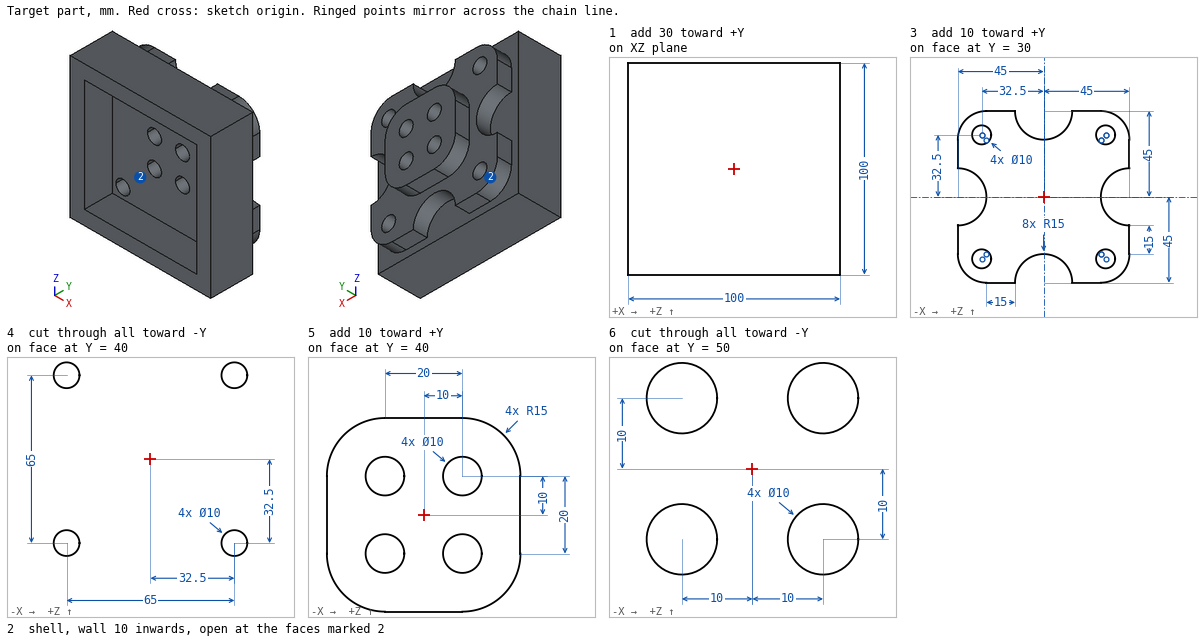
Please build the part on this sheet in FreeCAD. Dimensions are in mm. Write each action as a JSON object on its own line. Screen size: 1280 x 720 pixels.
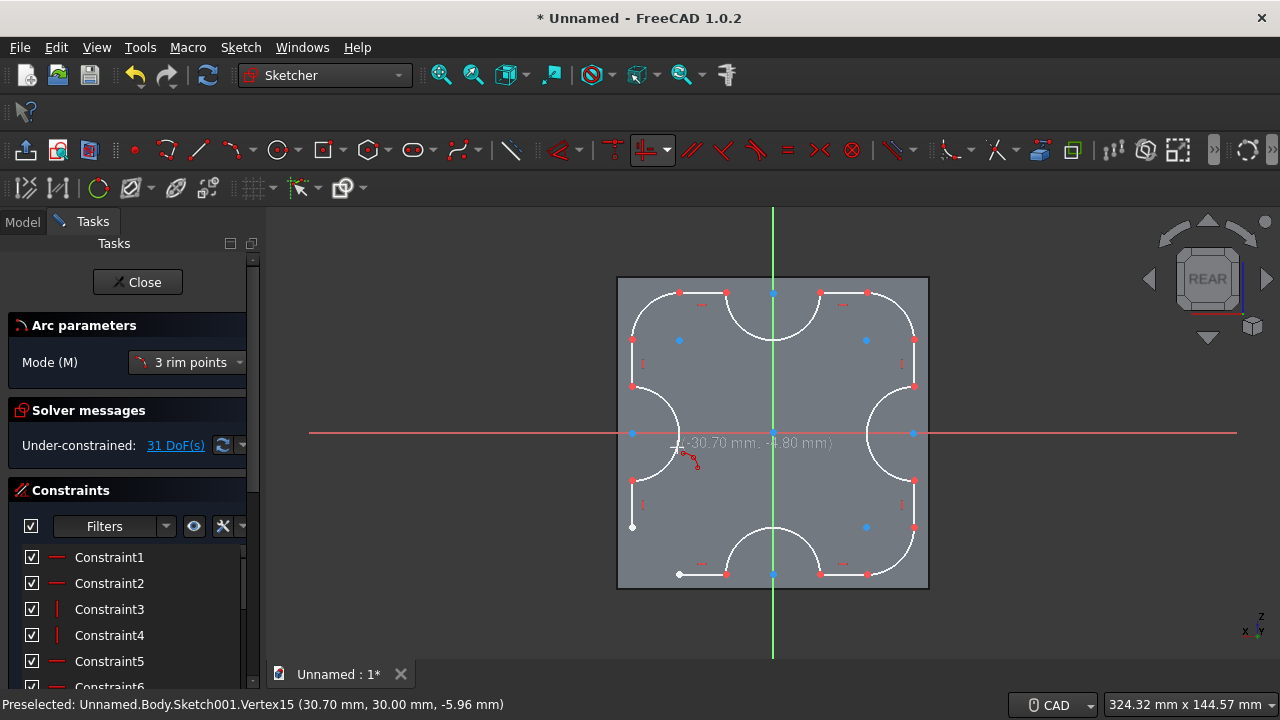
{"action": "left_click", "coordinate": [632, 528]}
{"action": "left_click", "coordinate": [679, 575]}
{"action": "left_click", "coordinate": [646, 560]}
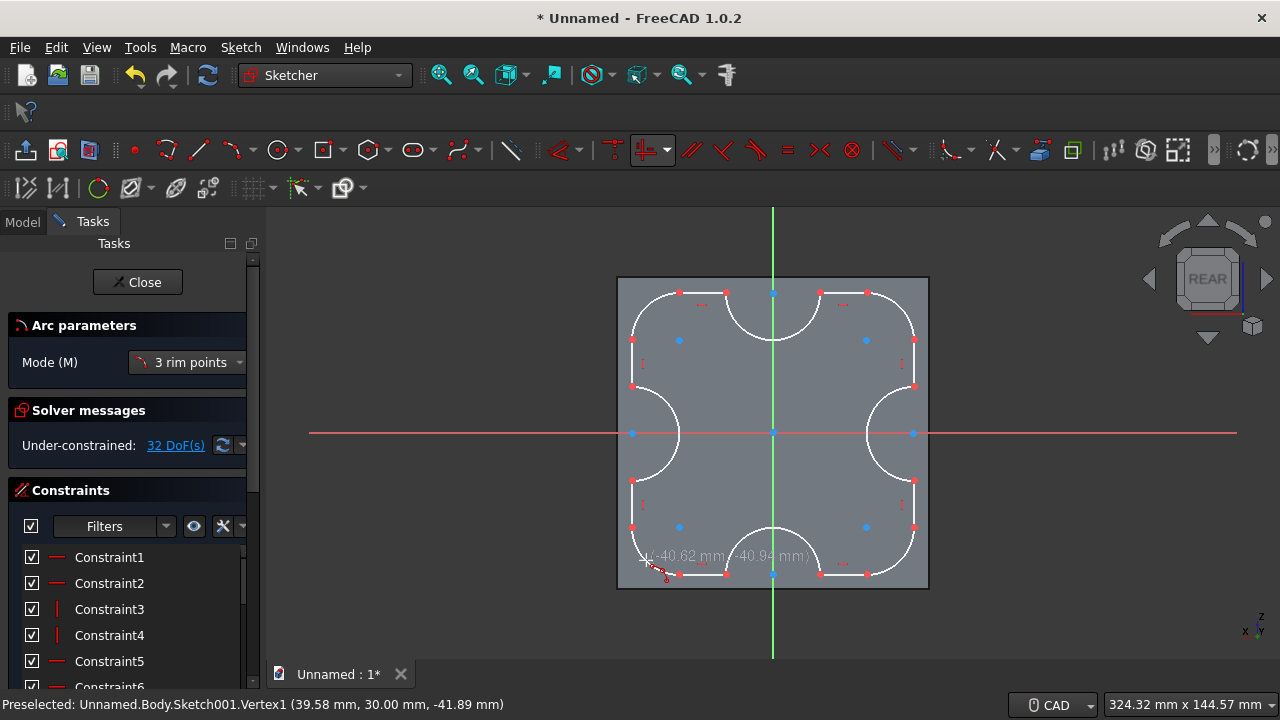
{"action": "left_click", "coordinate": [278, 150]}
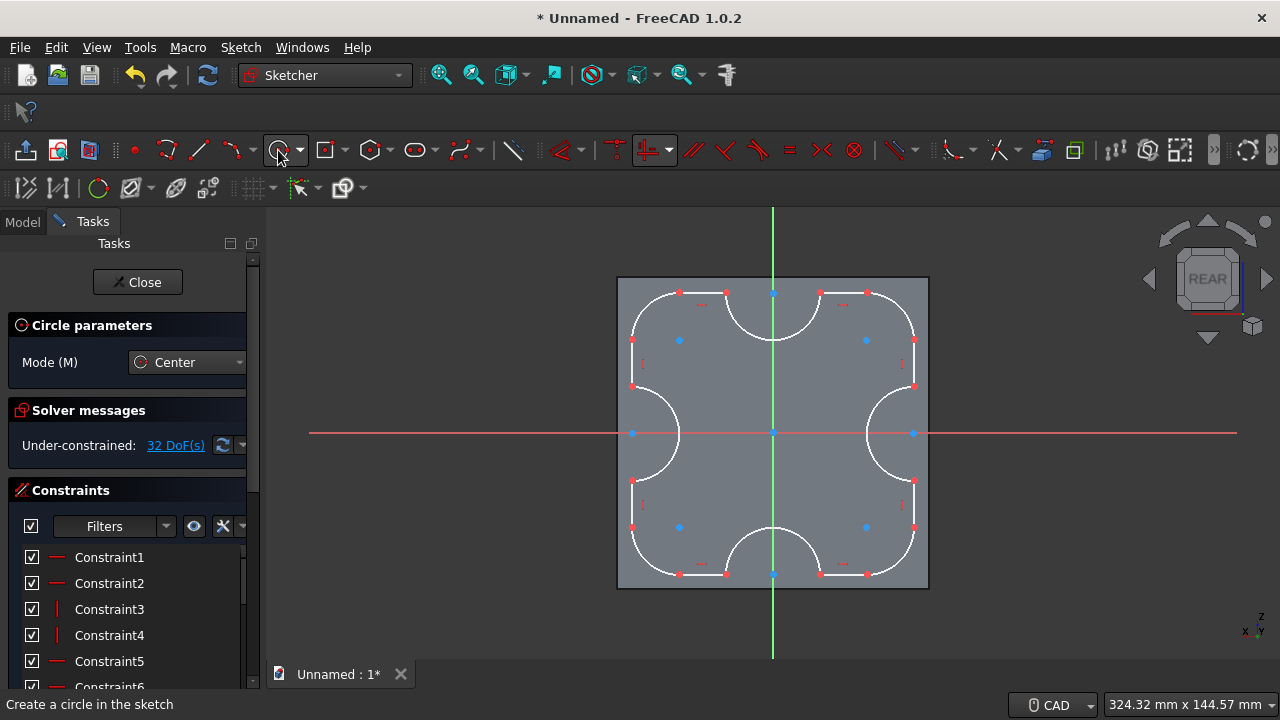
{"action": "scroll", "coordinate": [671, 331], "scroll_direction": "up", "scroll_amount": 2}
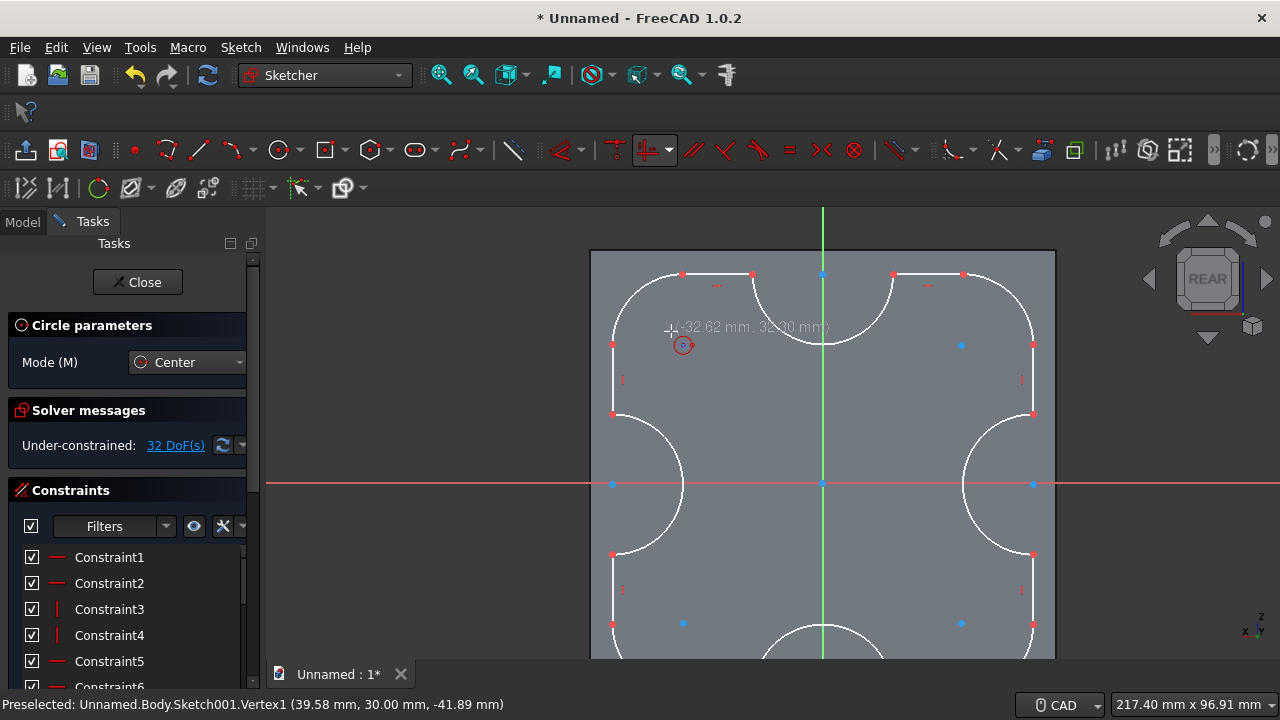
{"action": "left_click", "coordinate": [671, 331]}
{"action": "left_click", "coordinate": [688, 315]}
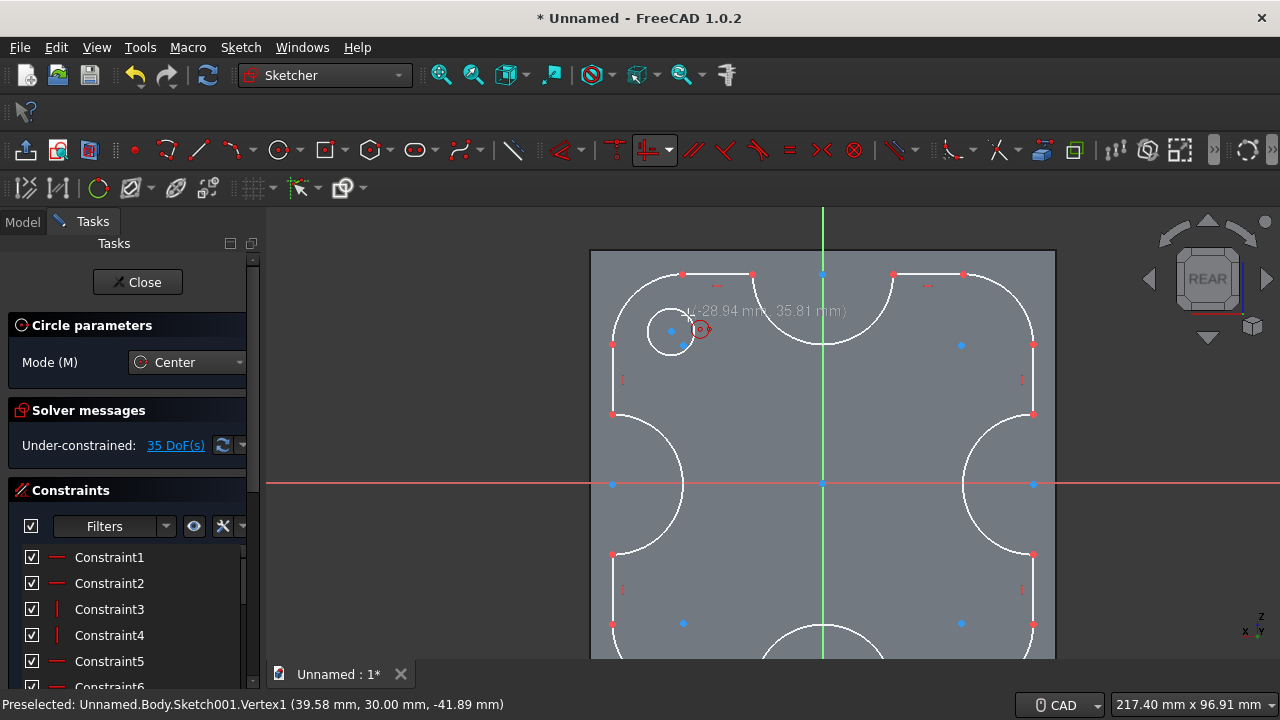
{"action": "left_click", "coordinate": [975, 331]}
{"action": "left_click", "coordinate": [991, 315]}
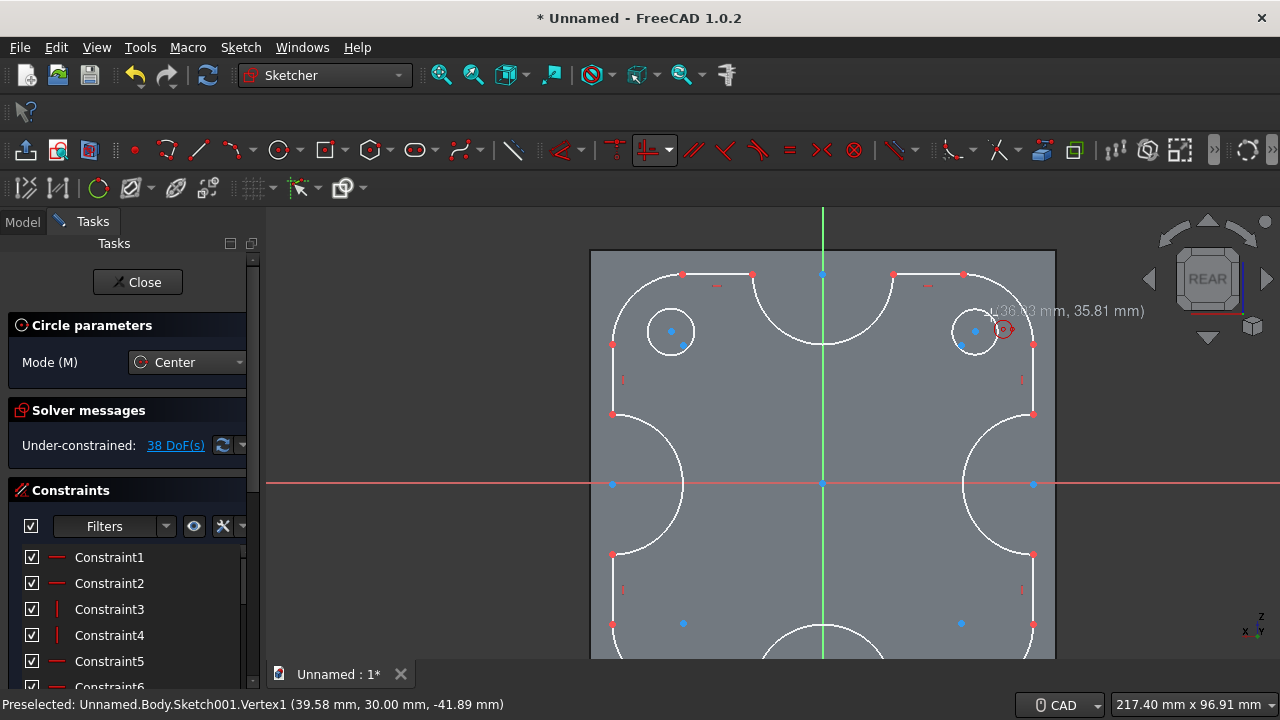
{"action": "scroll", "coordinate": [464, 331], "scroll_direction": "down", "scroll_amount": 2}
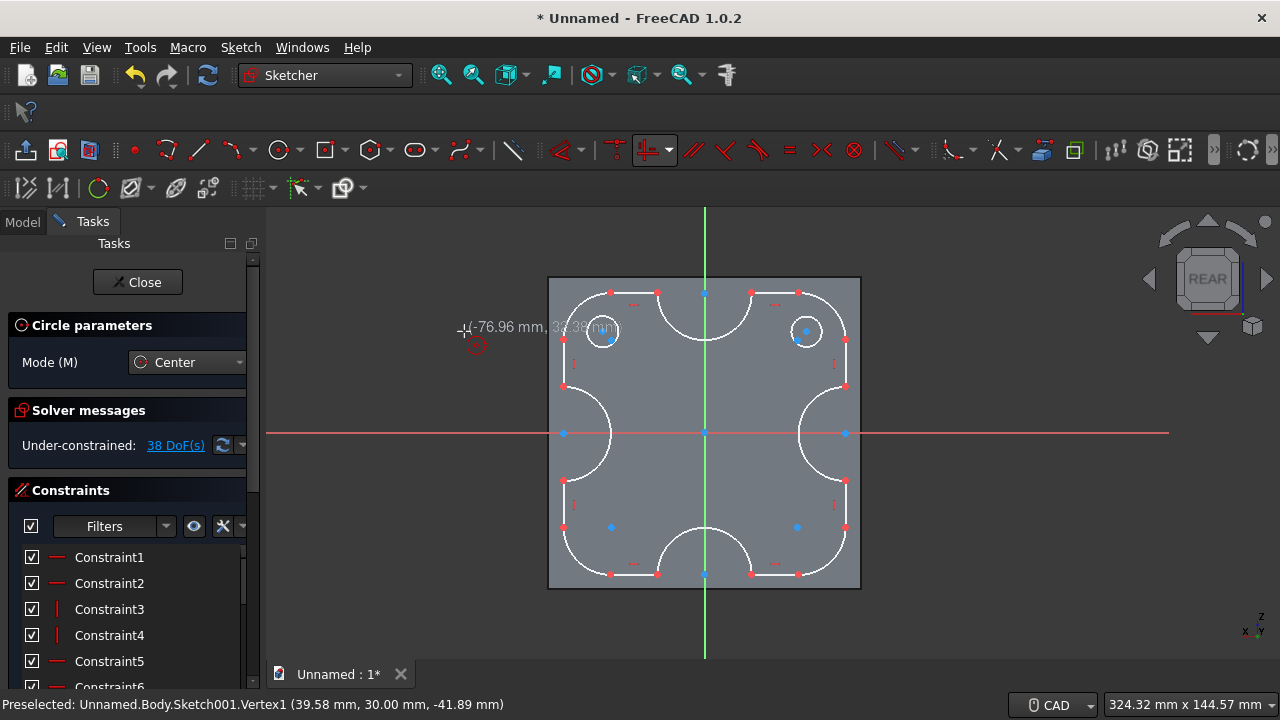
{"action": "scroll", "coordinate": [603, 535], "scroll_direction": "up", "scroll_amount": 2}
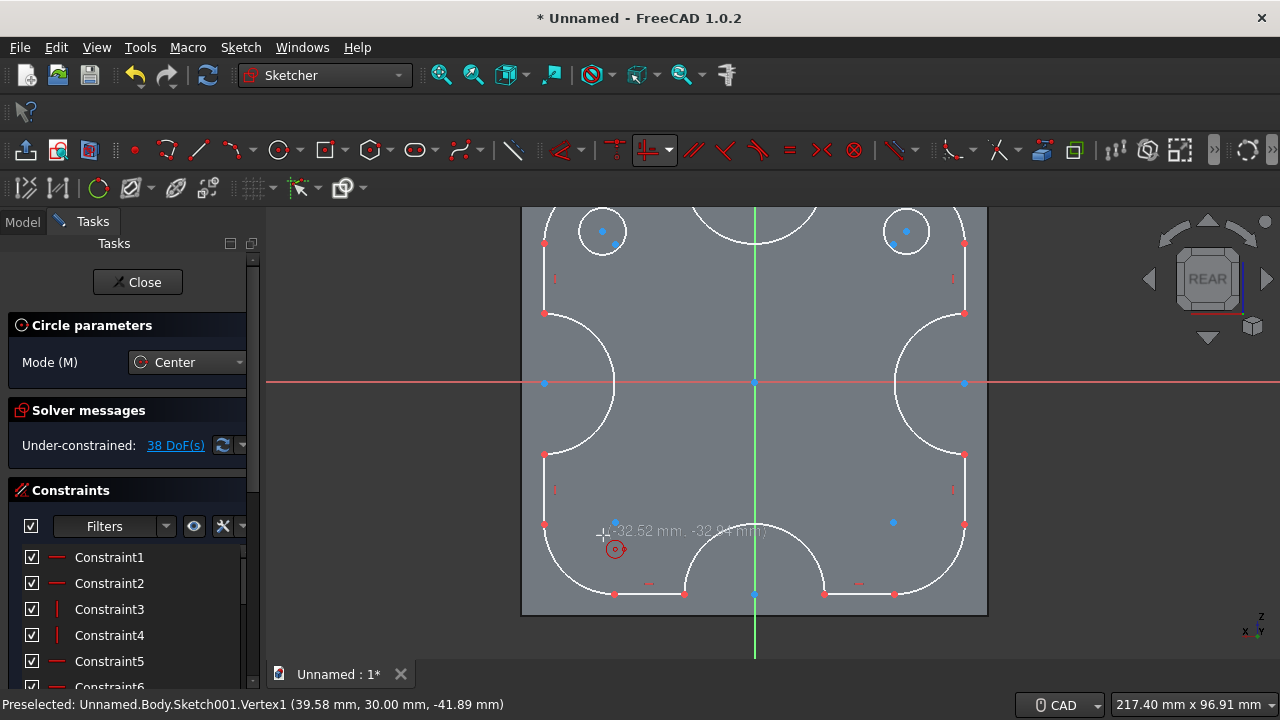
{"action": "left_click", "coordinate": [603, 534]}
{"action": "left_click", "coordinate": [586, 518]}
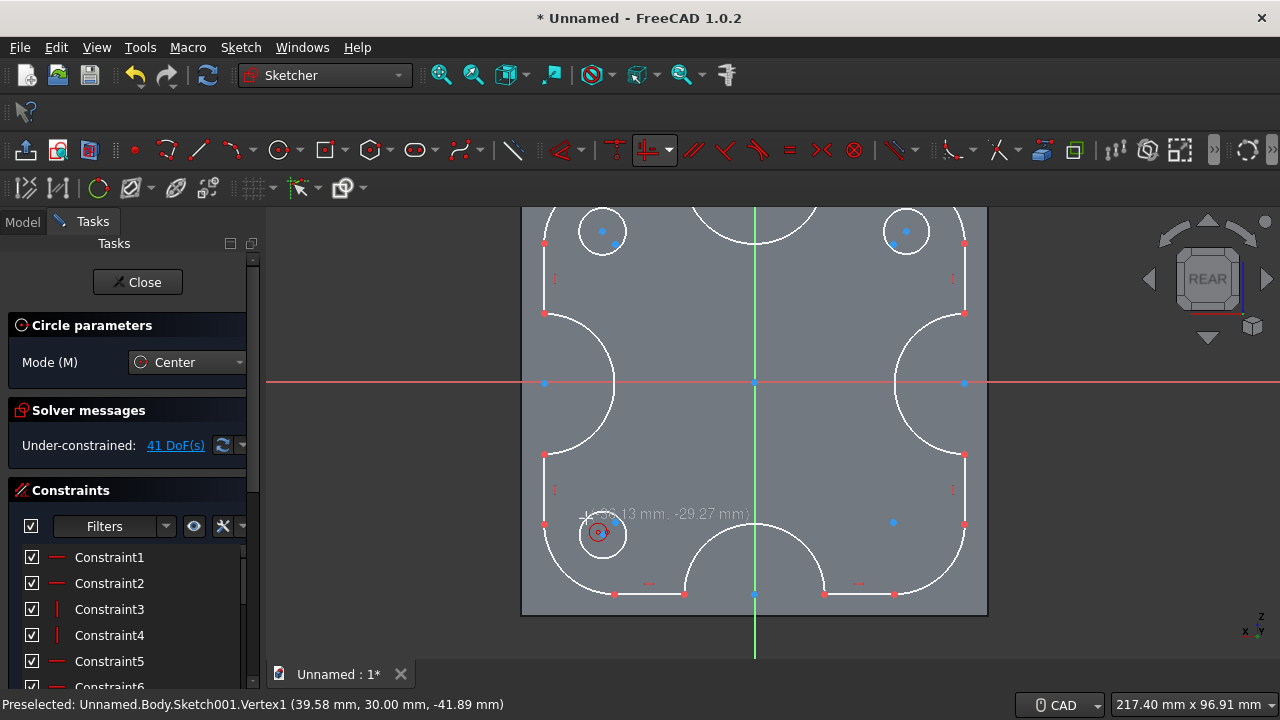
{"action": "left_click", "coordinate": [906, 534]}
{"action": "left_click", "coordinate": [923, 518]}
{"action": "key", "text": "Escape"}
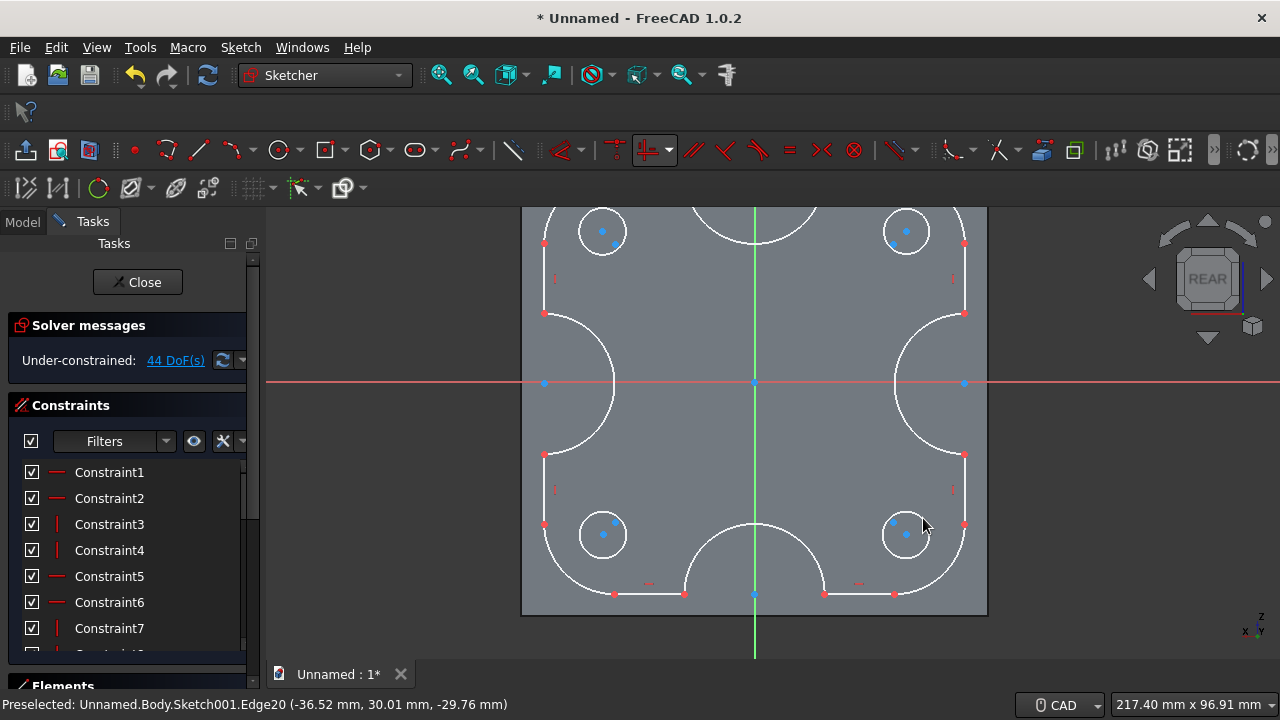
{"action": "left_click", "coordinate": [635, 594]}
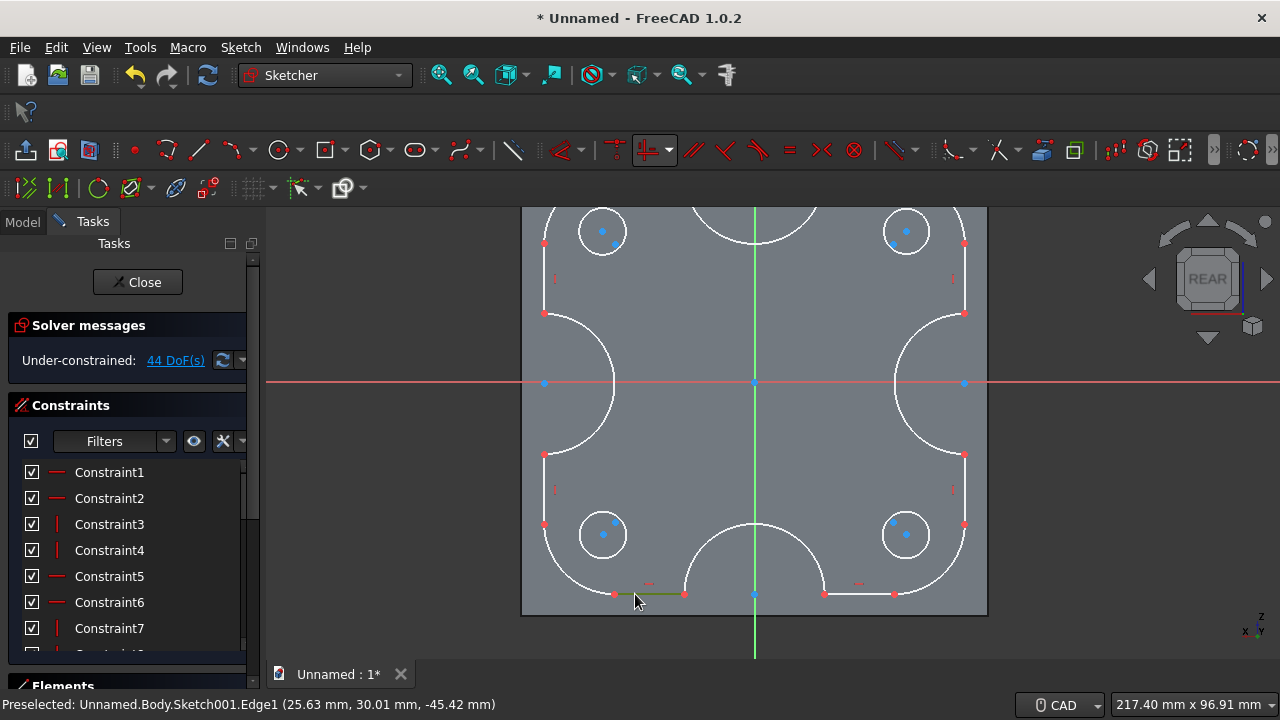
{"action": "left_click", "coordinate": [552, 556]}